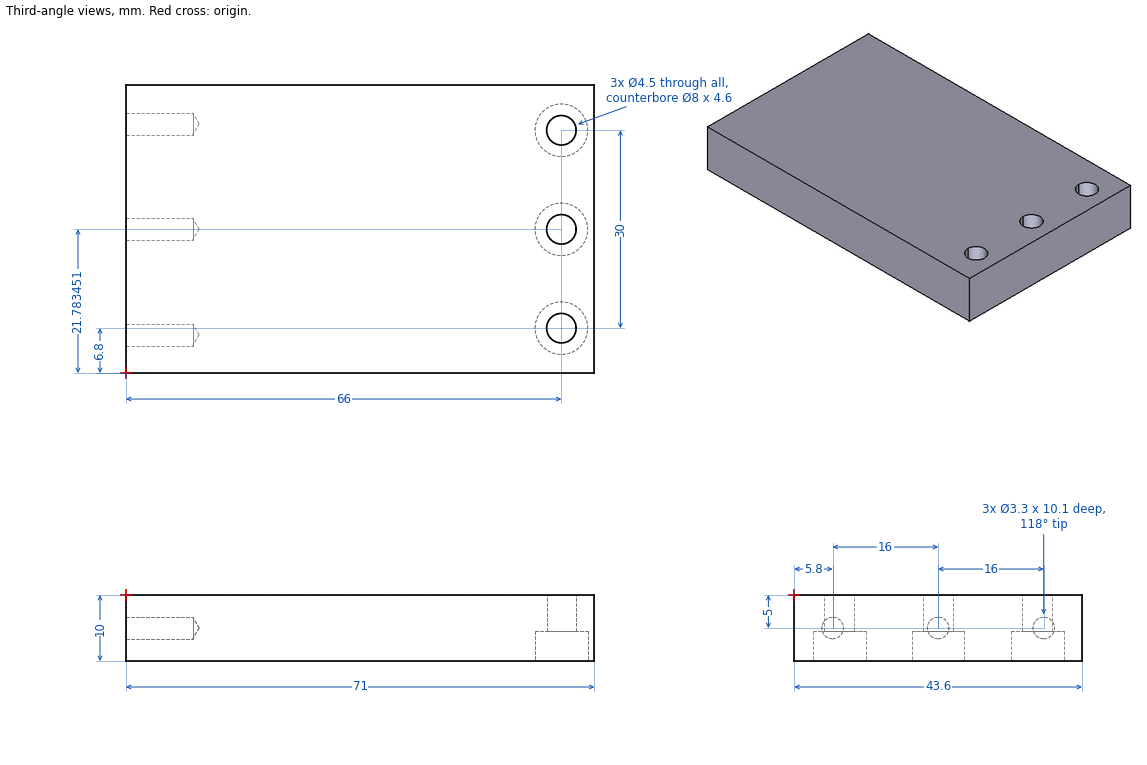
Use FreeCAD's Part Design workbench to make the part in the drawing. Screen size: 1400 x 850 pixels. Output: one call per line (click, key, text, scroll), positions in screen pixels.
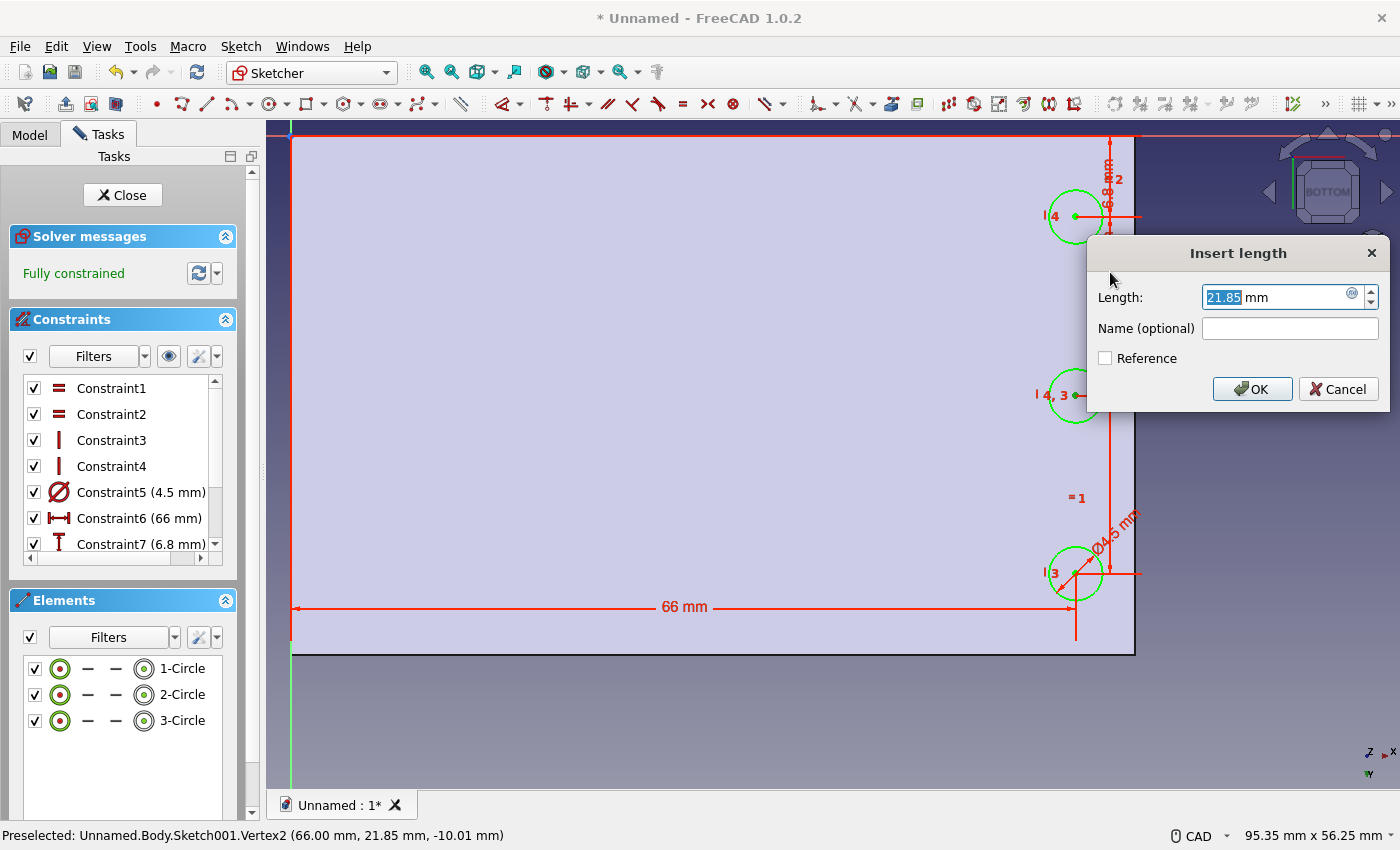
text(21.783451)
key(Return)
key(Escape)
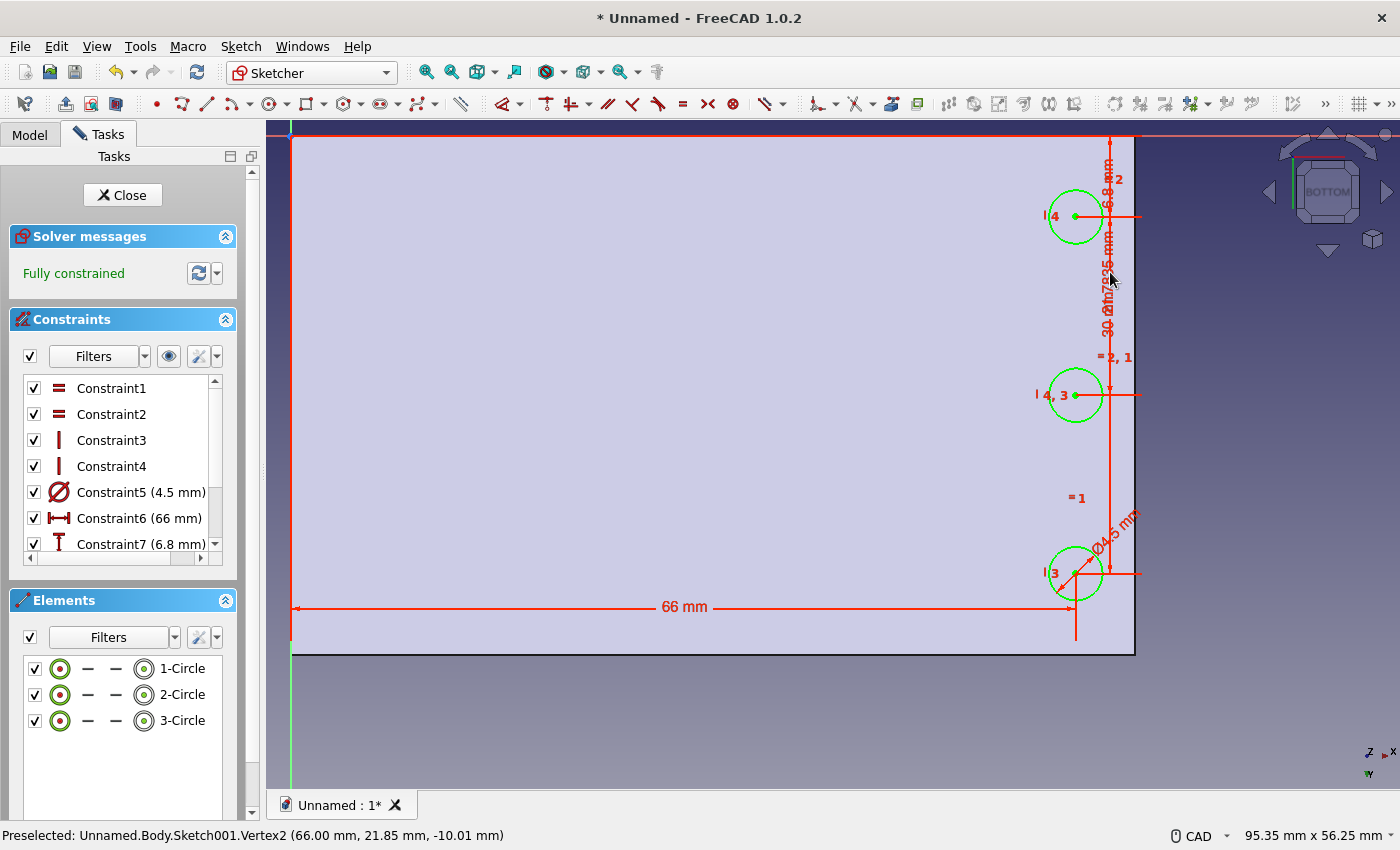
click(123, 195)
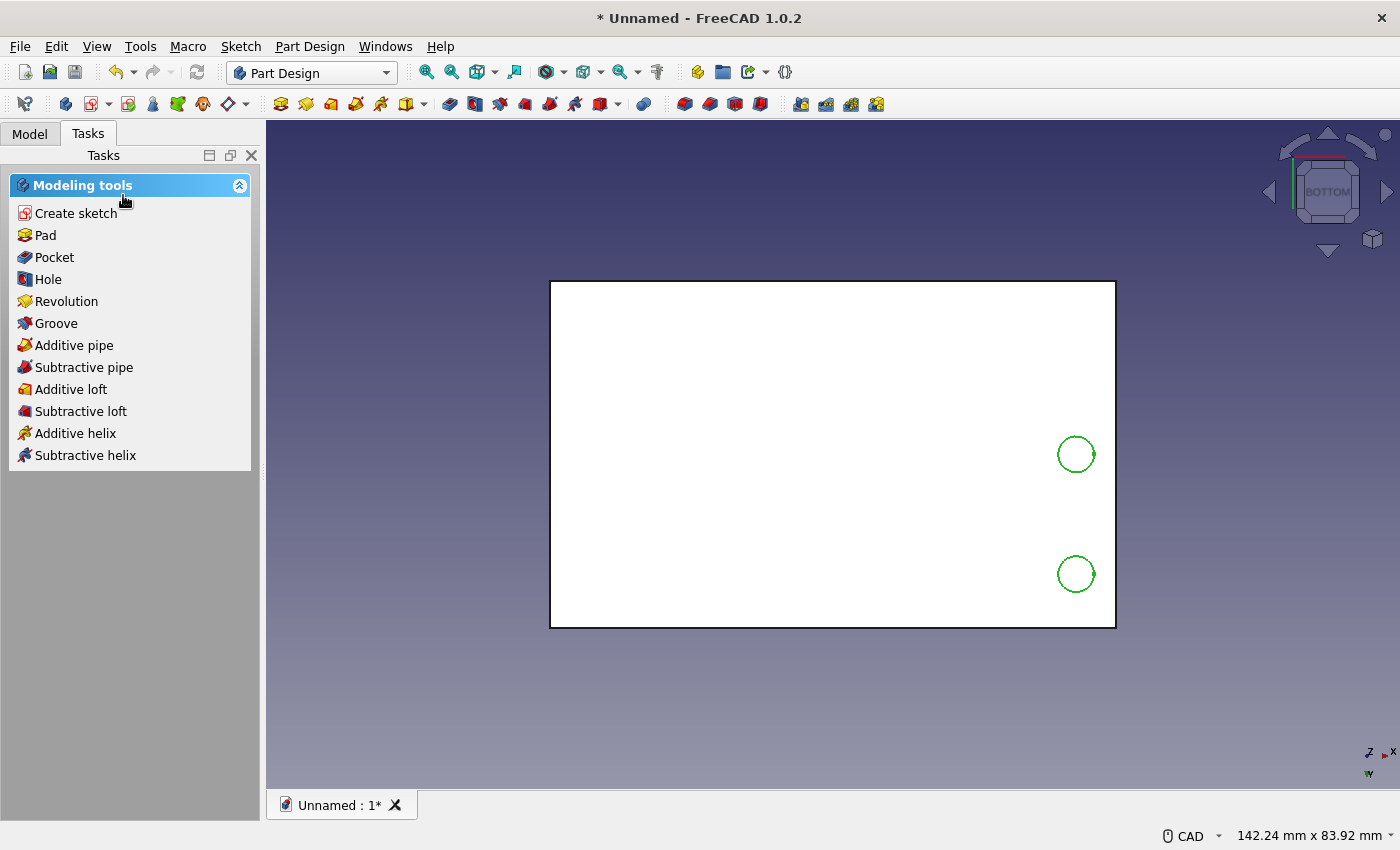
click(475, 104)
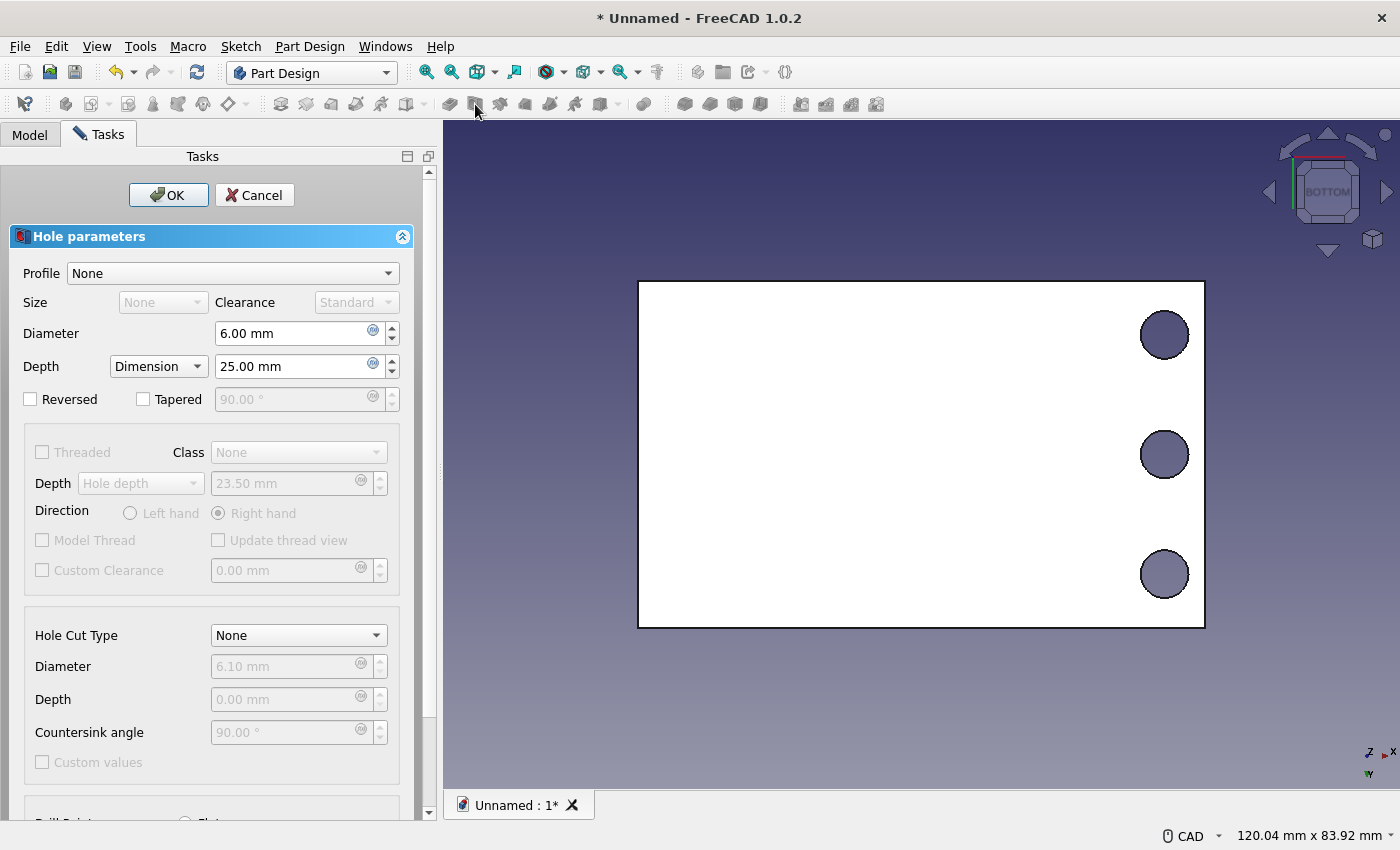
triple_click(300, 334)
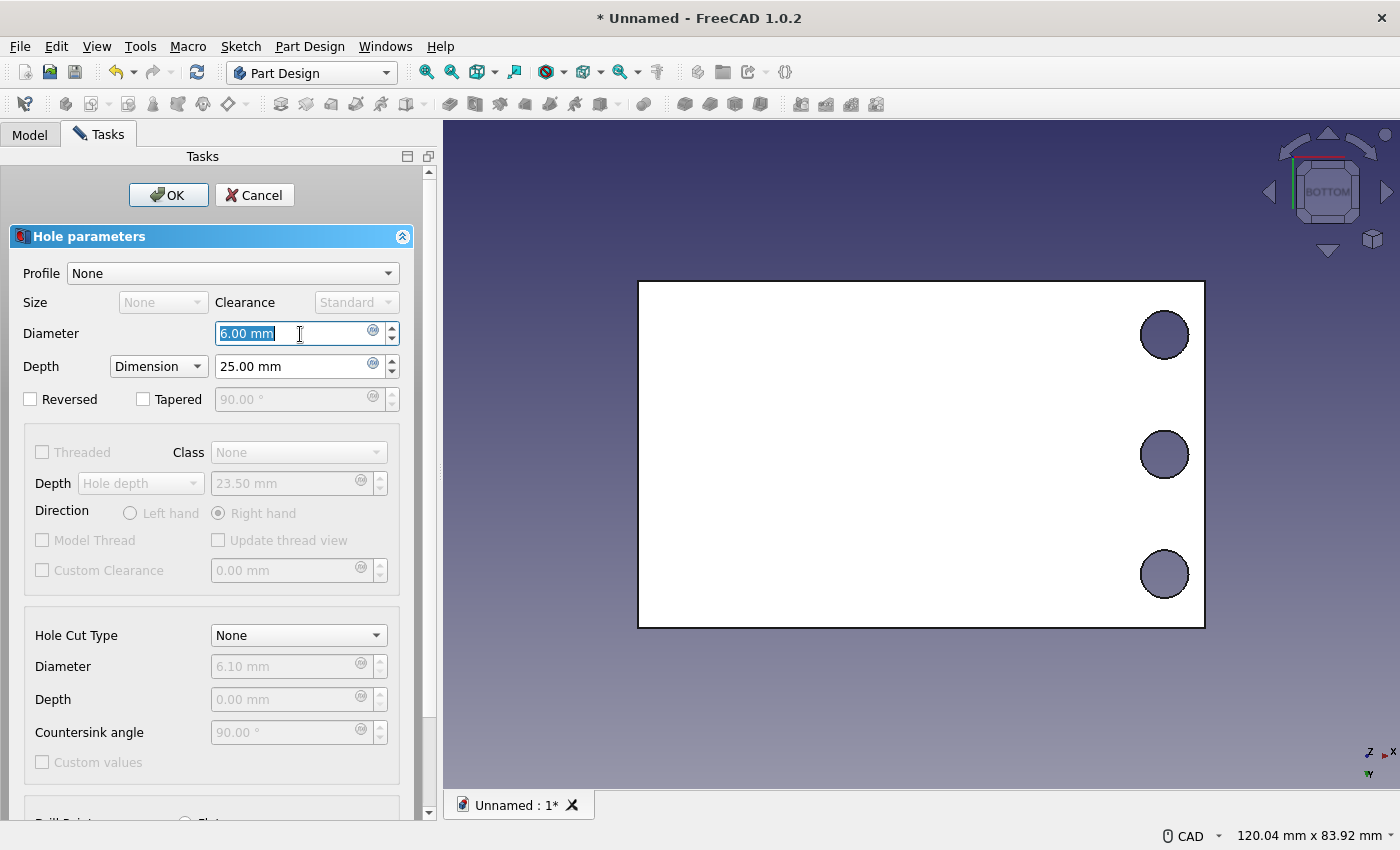
text(4.5)
key(Tab)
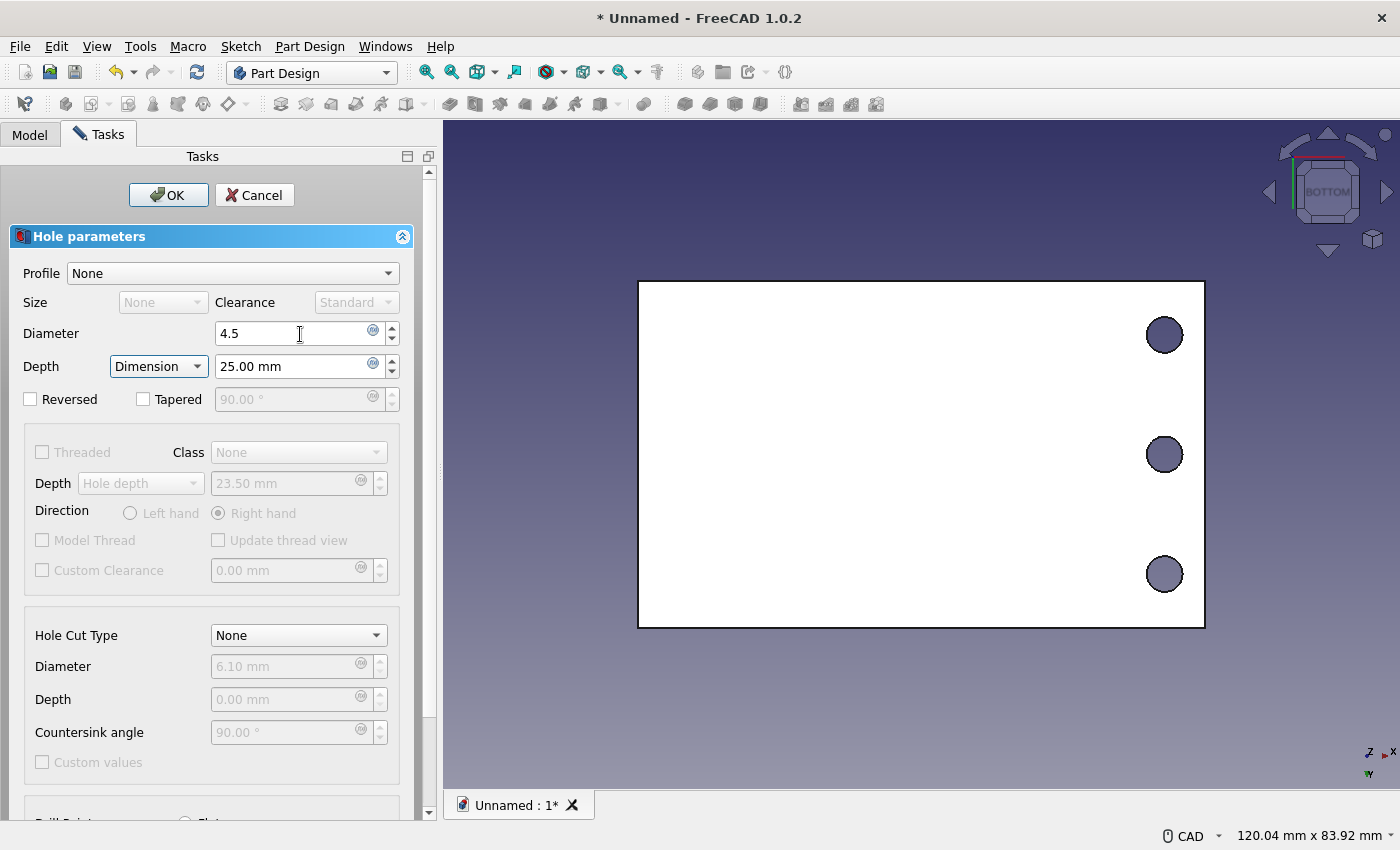
click(160, 366)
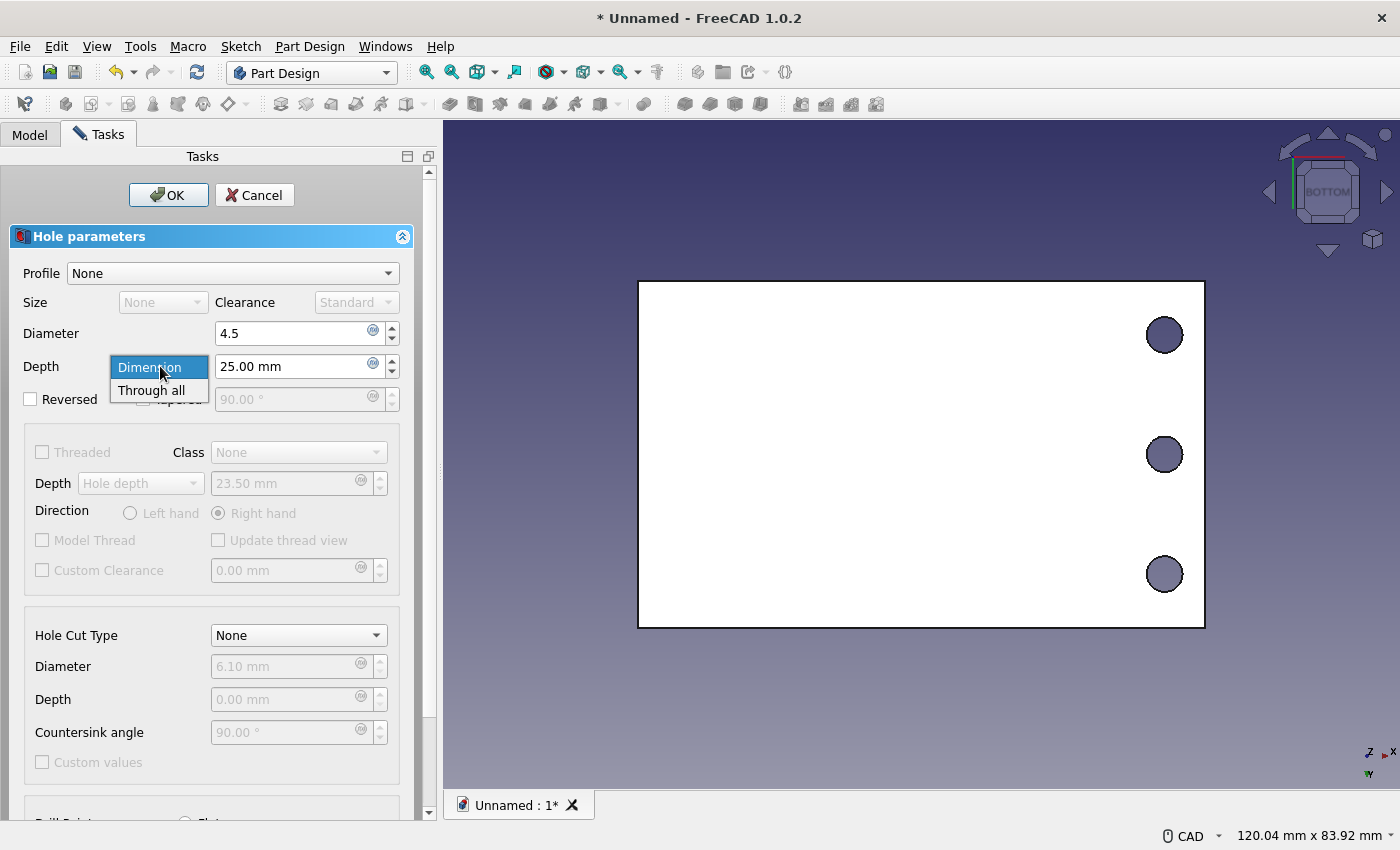
click(158, 390)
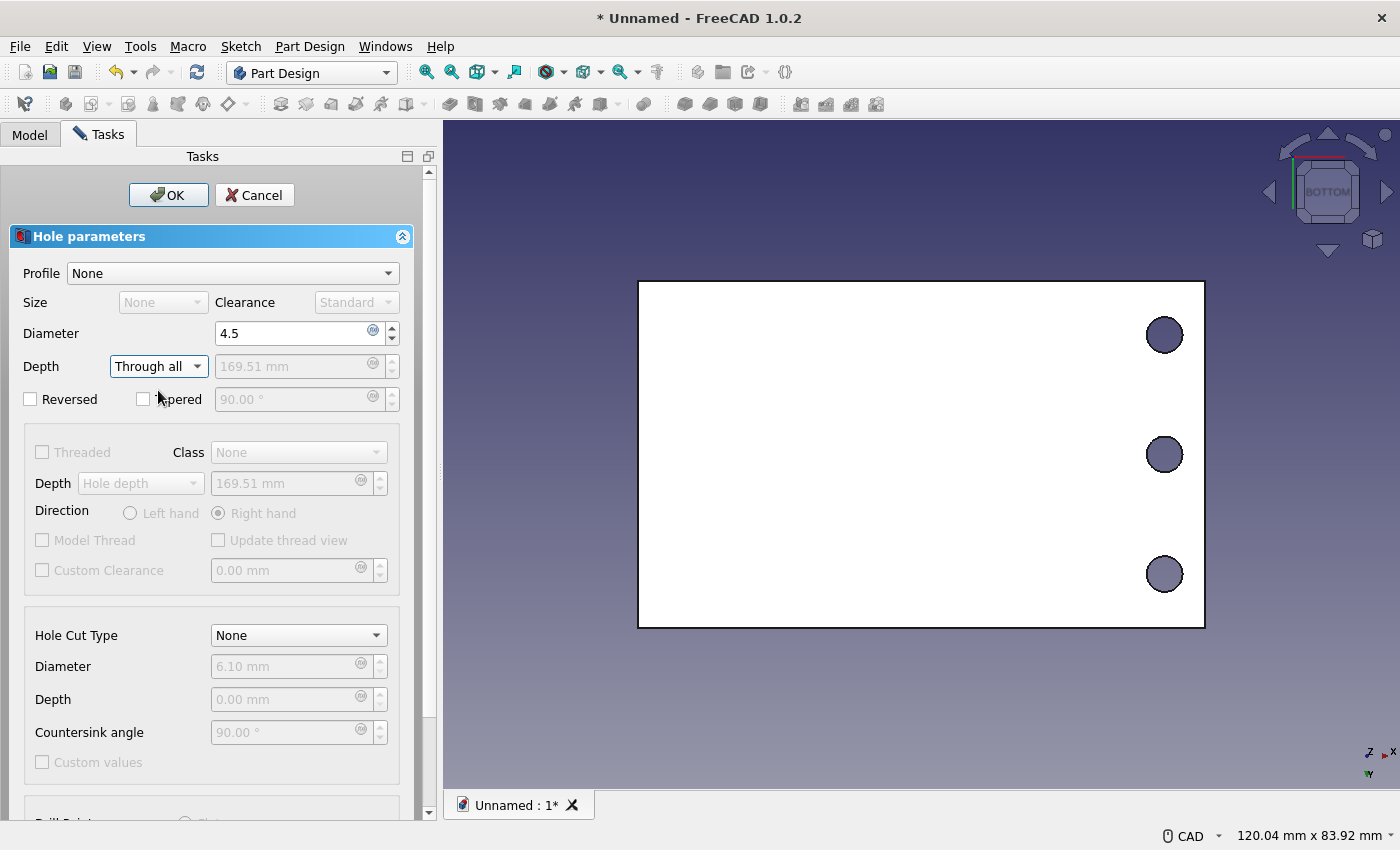
click(300, 636)